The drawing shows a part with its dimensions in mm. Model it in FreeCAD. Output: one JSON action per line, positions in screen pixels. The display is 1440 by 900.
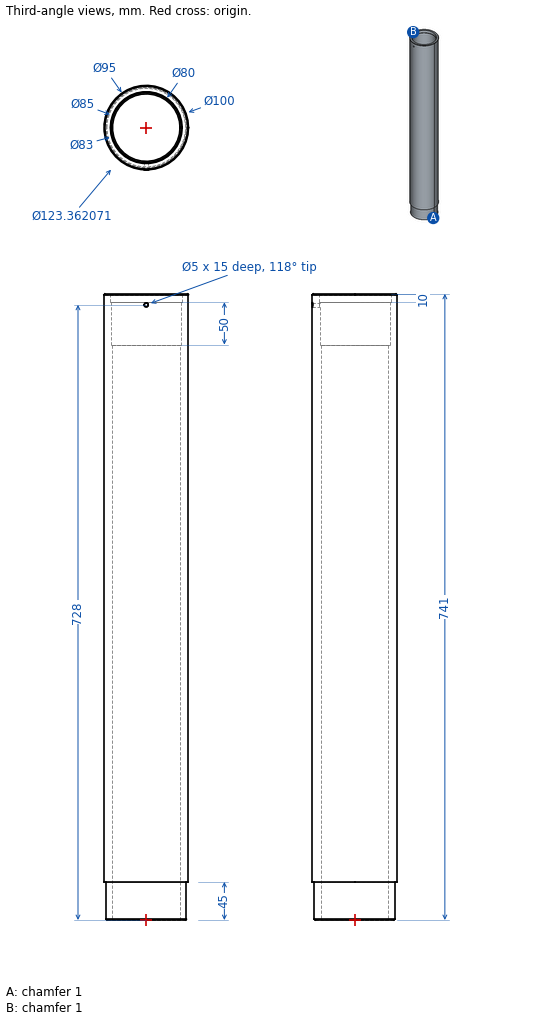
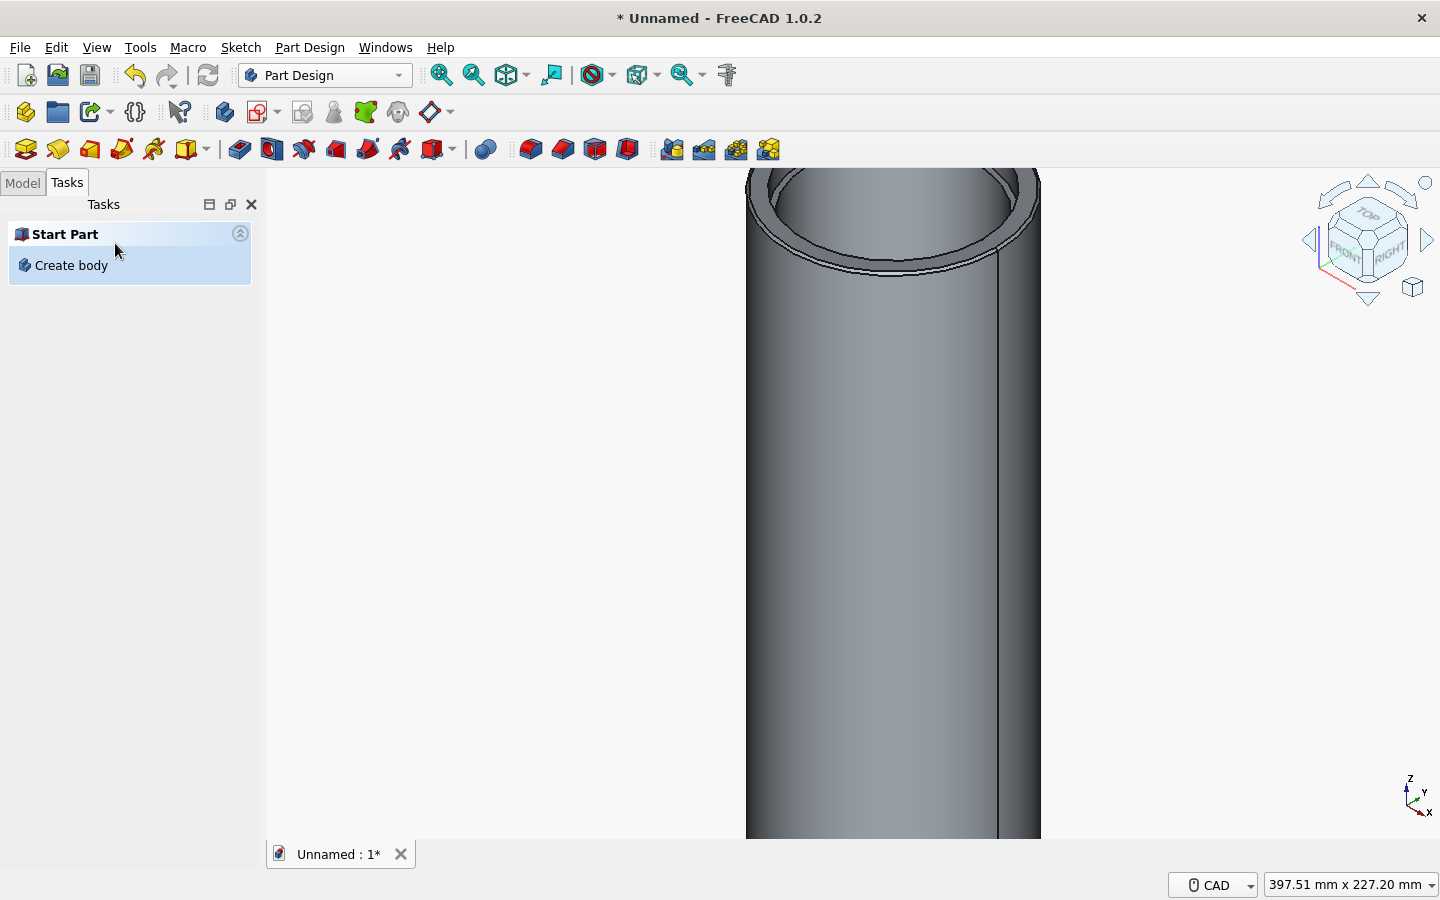
{"action": "left_click", "coordinate": [442, 76]}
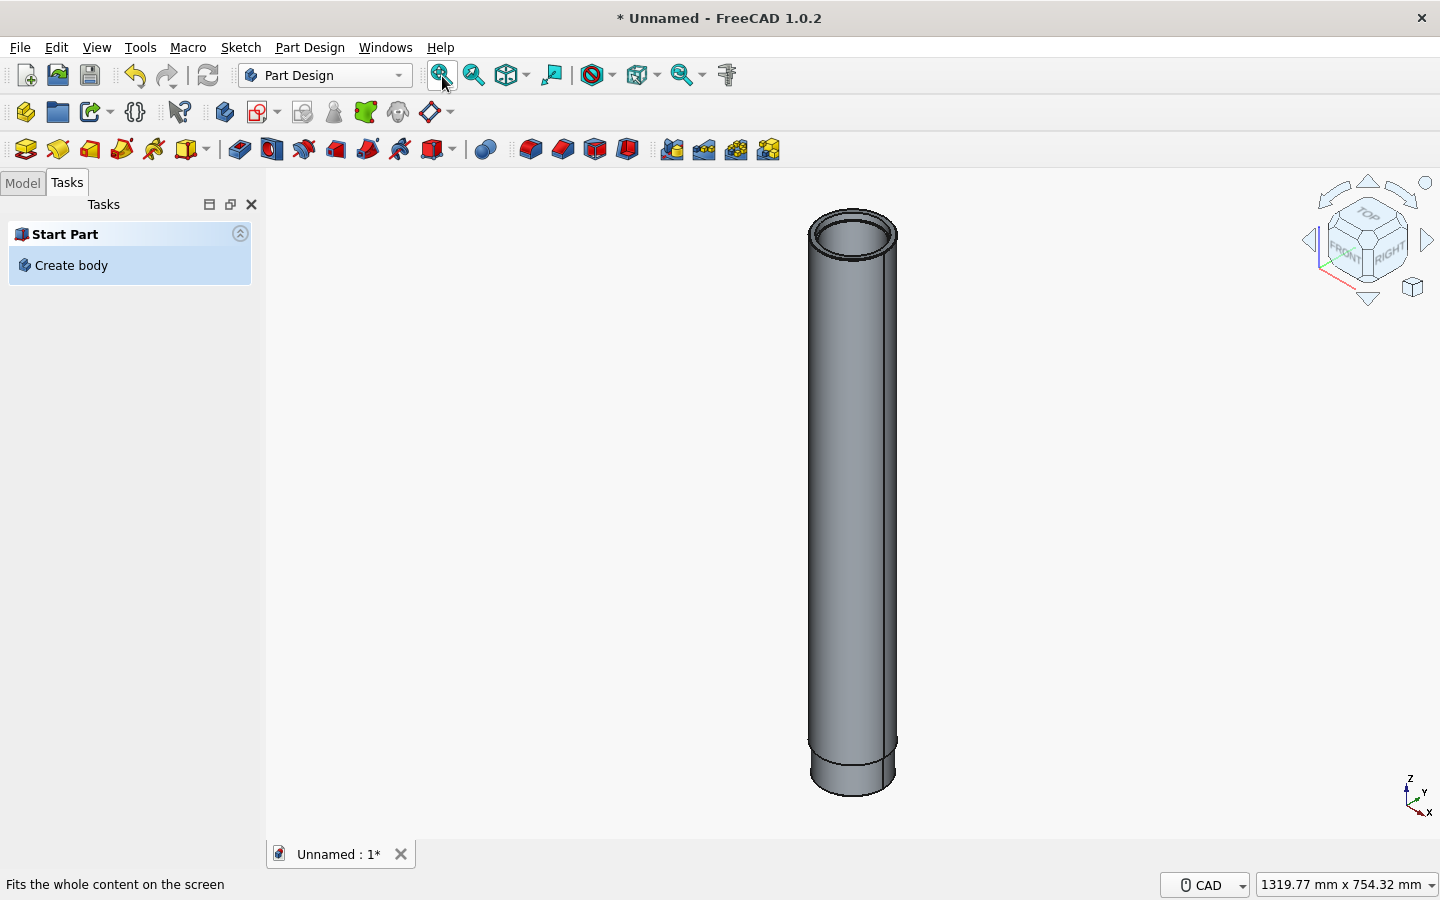
{"action": "scroll", "coordinate": [821, 229], "scroll_direction": "up", "scroll_amount": 14}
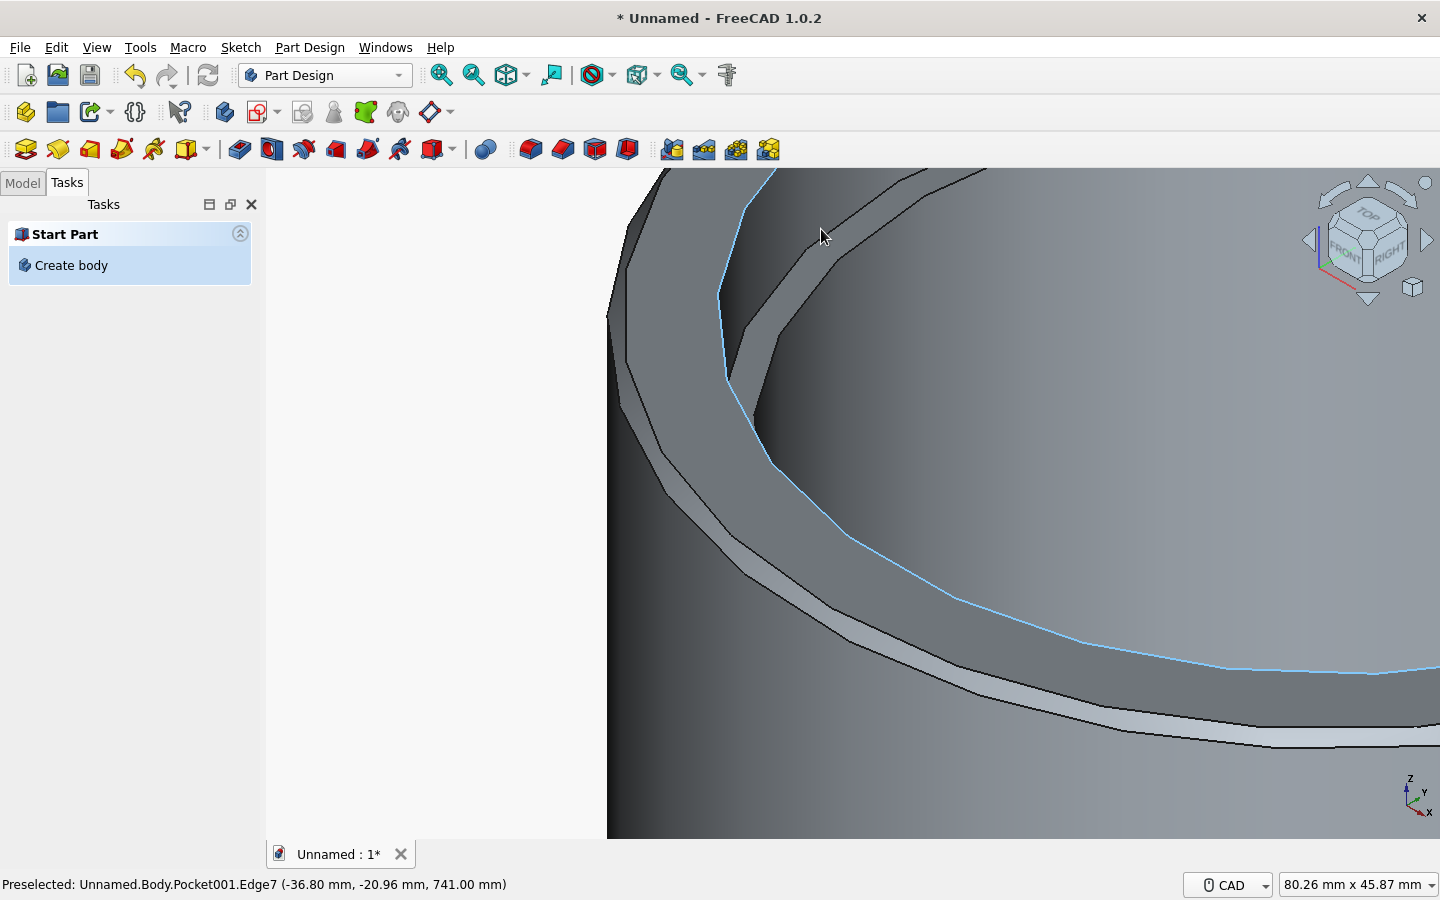
{"action": "left_click", "coordinate": [820, 249]}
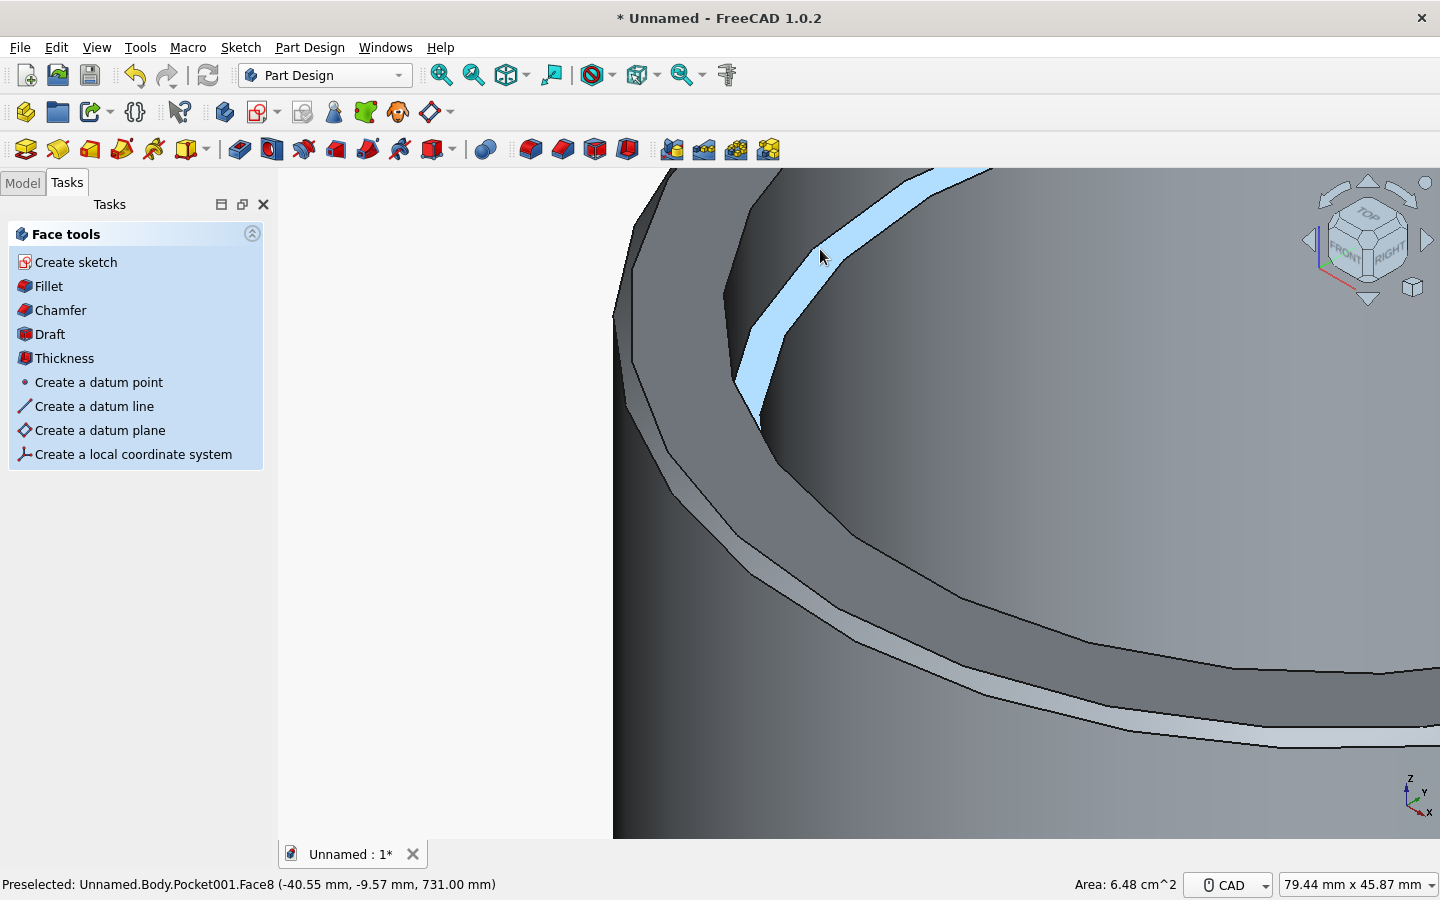
{"action": "left_click", "coordinate": [258, 112]}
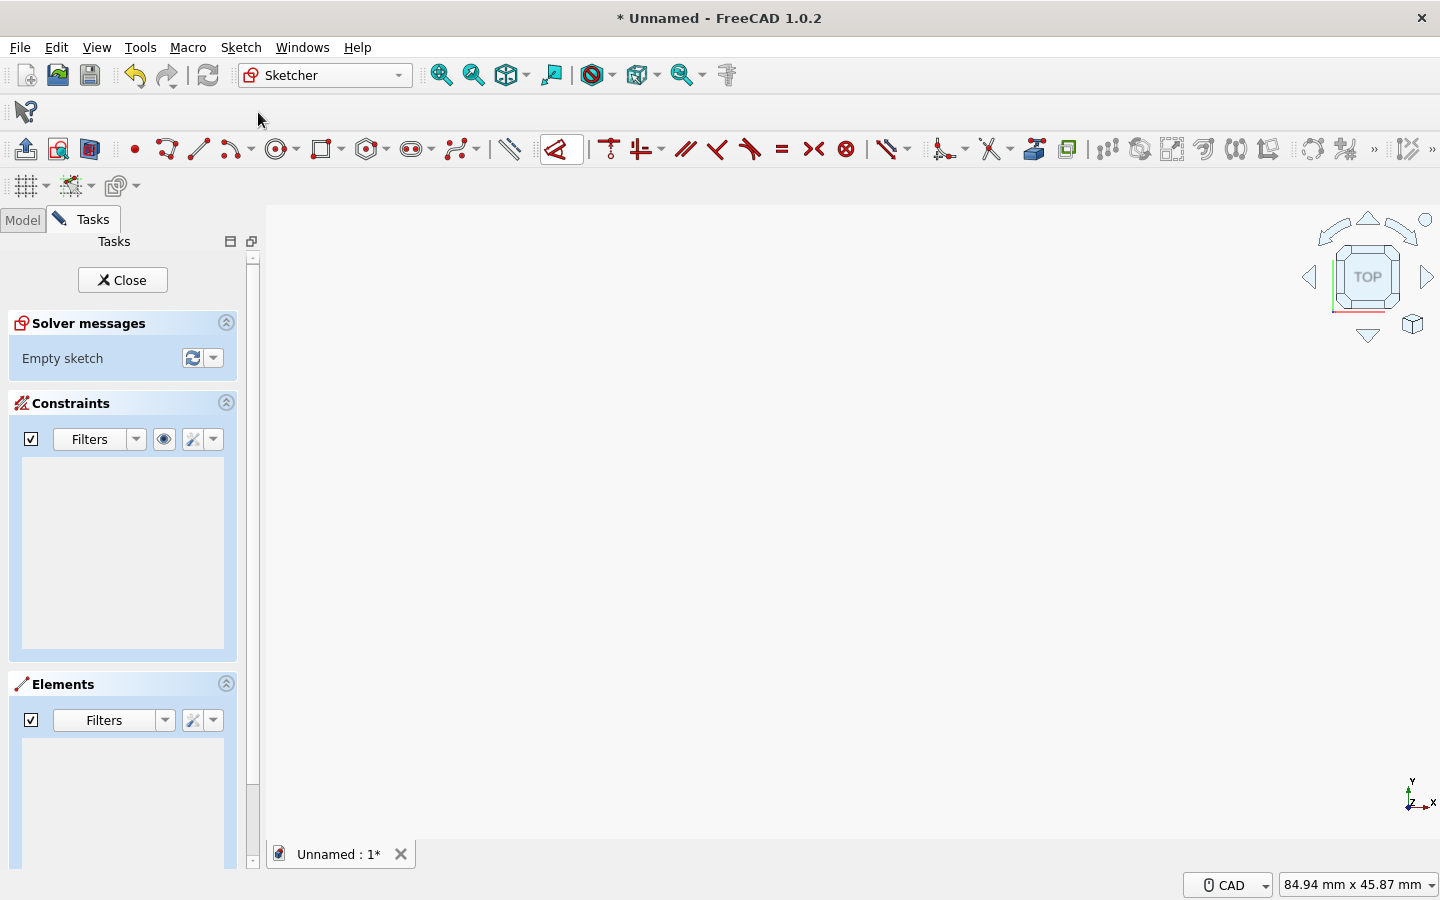
{"action": "scroll", "coordinate": [294, 233], "scroll_direction": "down", "scroll_amount": 7}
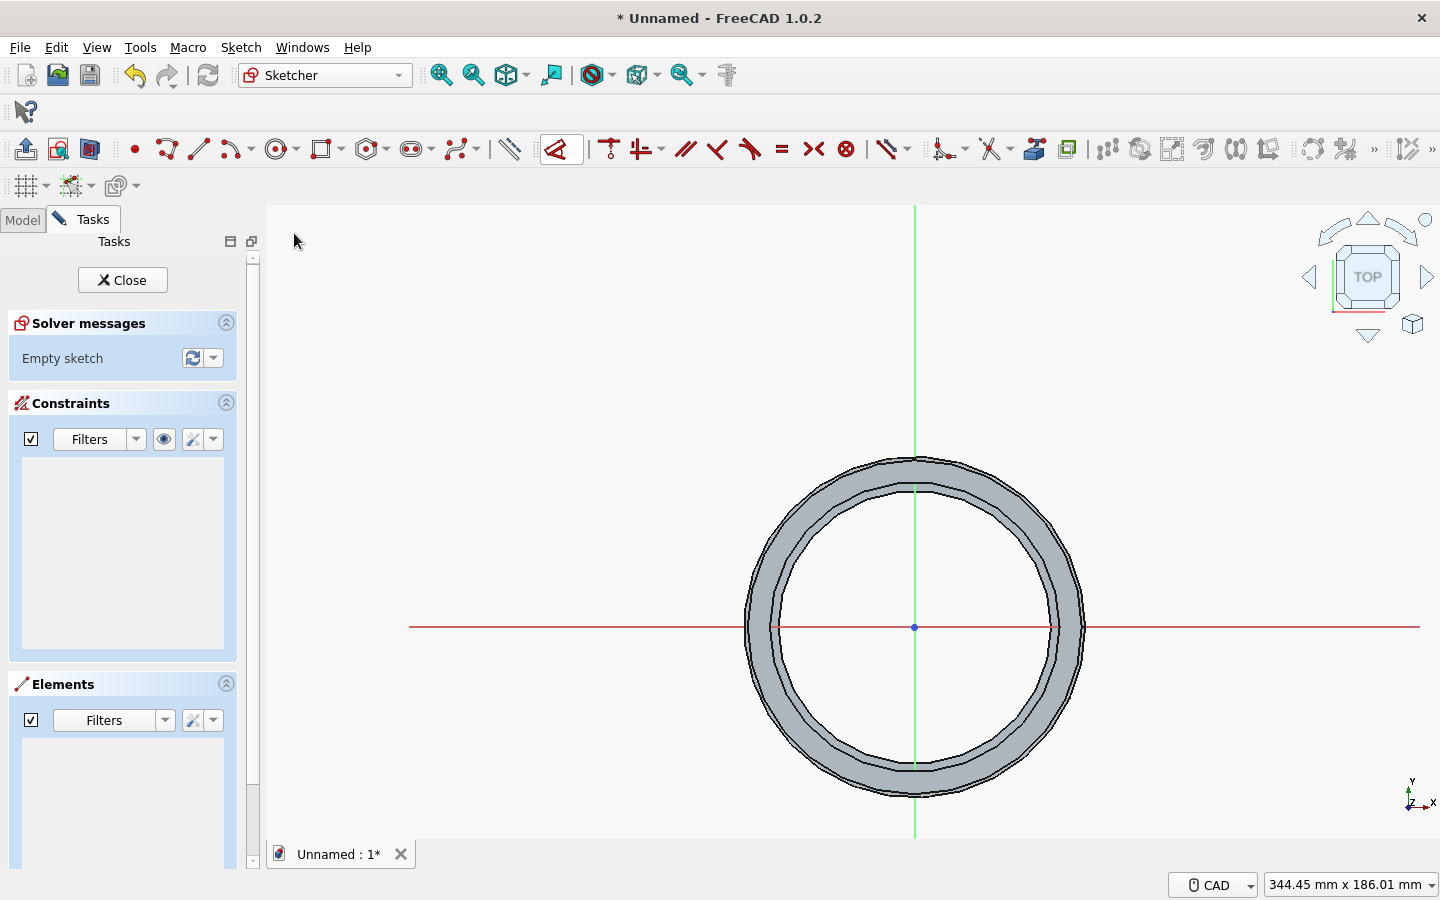
{"action": "scroll", "coordinate": [1180, 811], "scroll_direction": "up", "scroll_amount": 2}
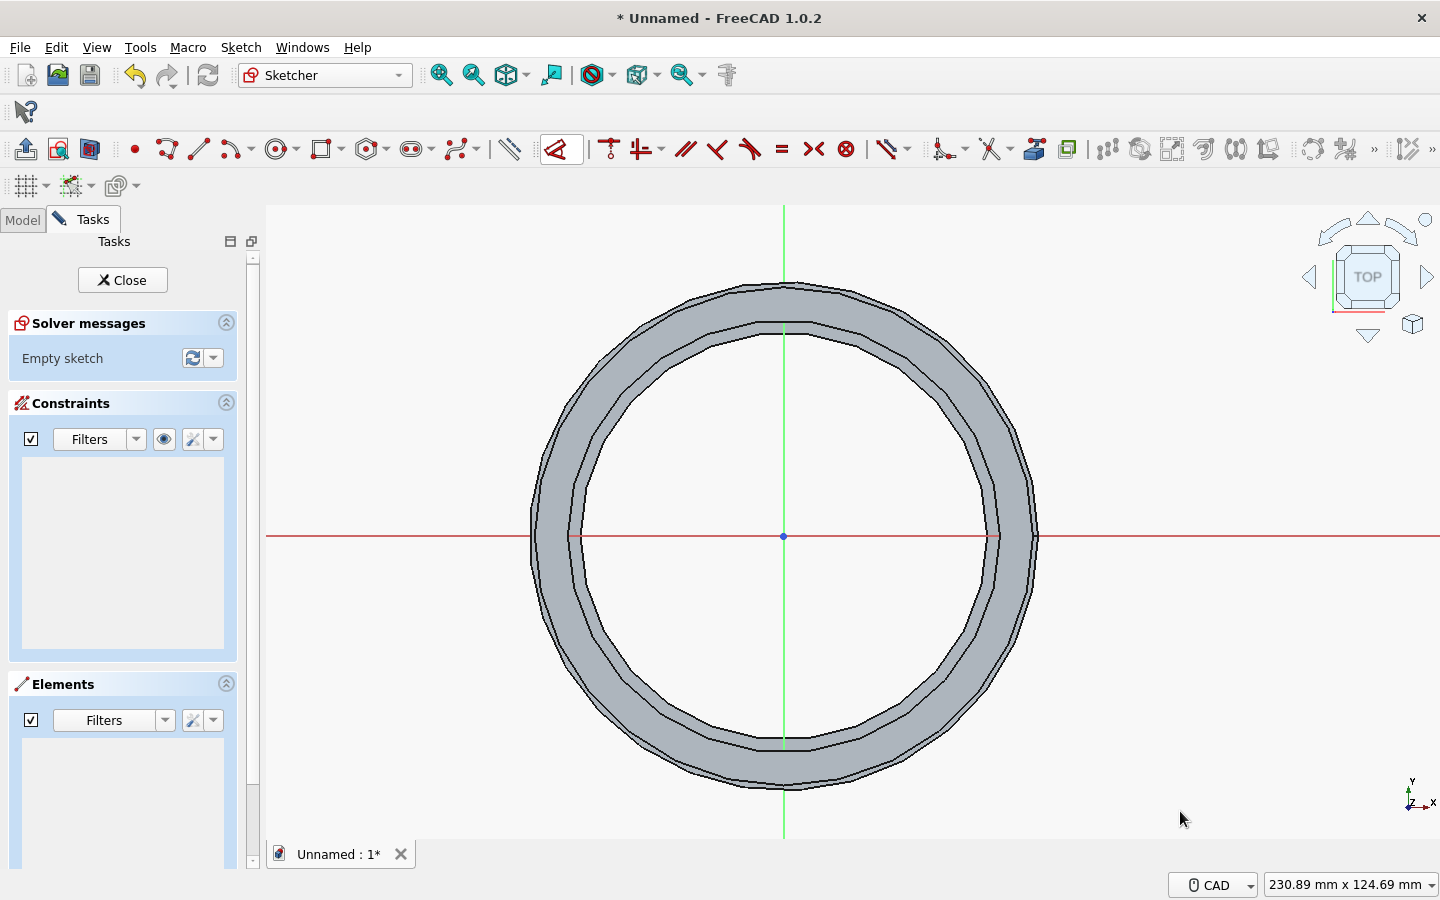
{"action": "left_click", "coordinate": [276, 150]}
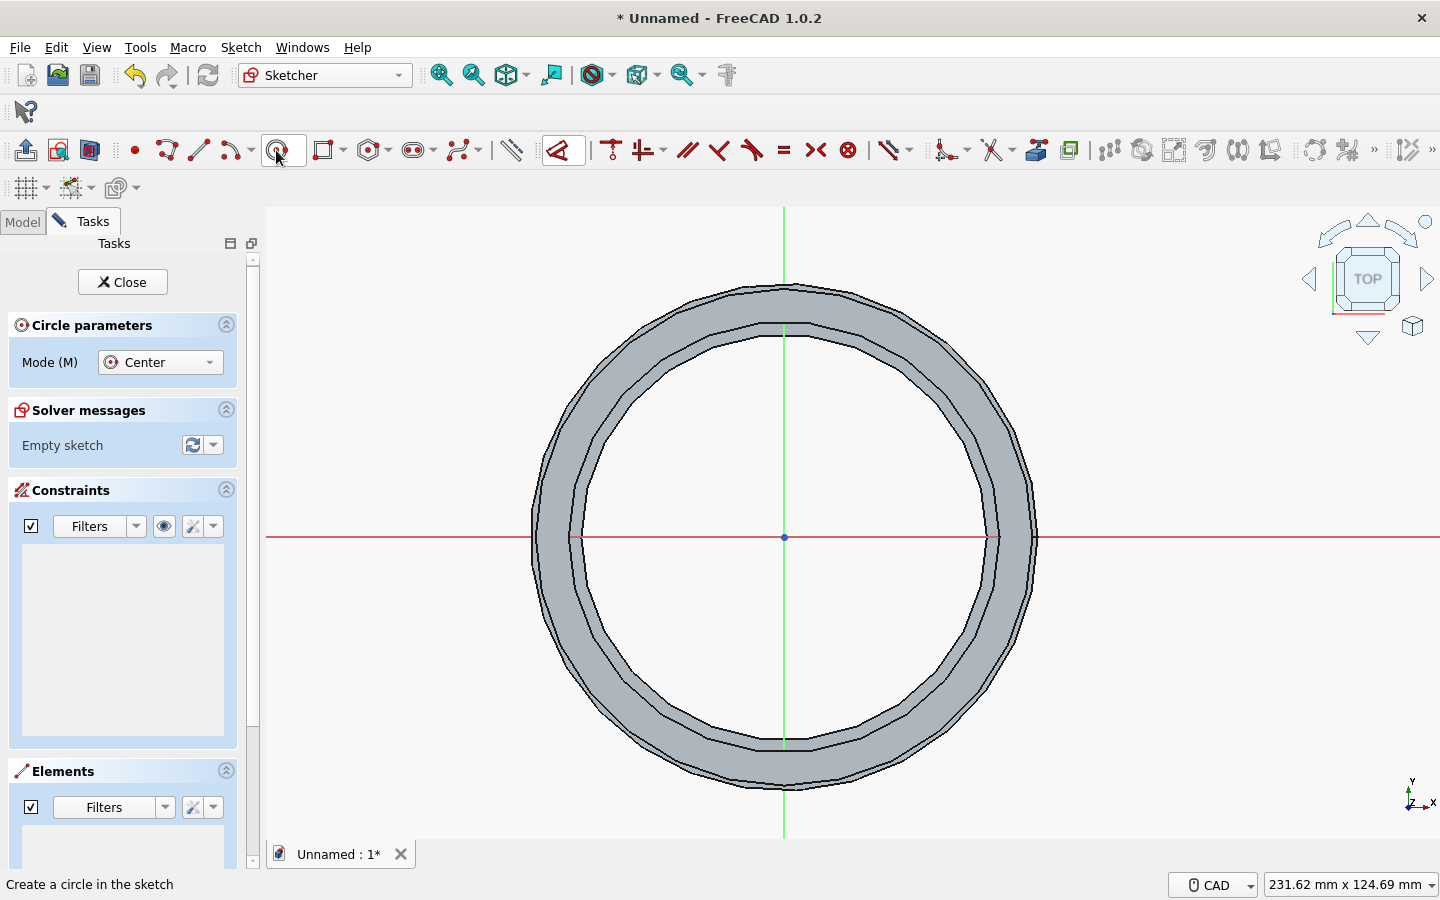
{"action": "left_click", "coordinate": [784, 537]}
{"action": "left_click", "coordinate": [933, 389]}
{"action": "key", "text": "Escape"}